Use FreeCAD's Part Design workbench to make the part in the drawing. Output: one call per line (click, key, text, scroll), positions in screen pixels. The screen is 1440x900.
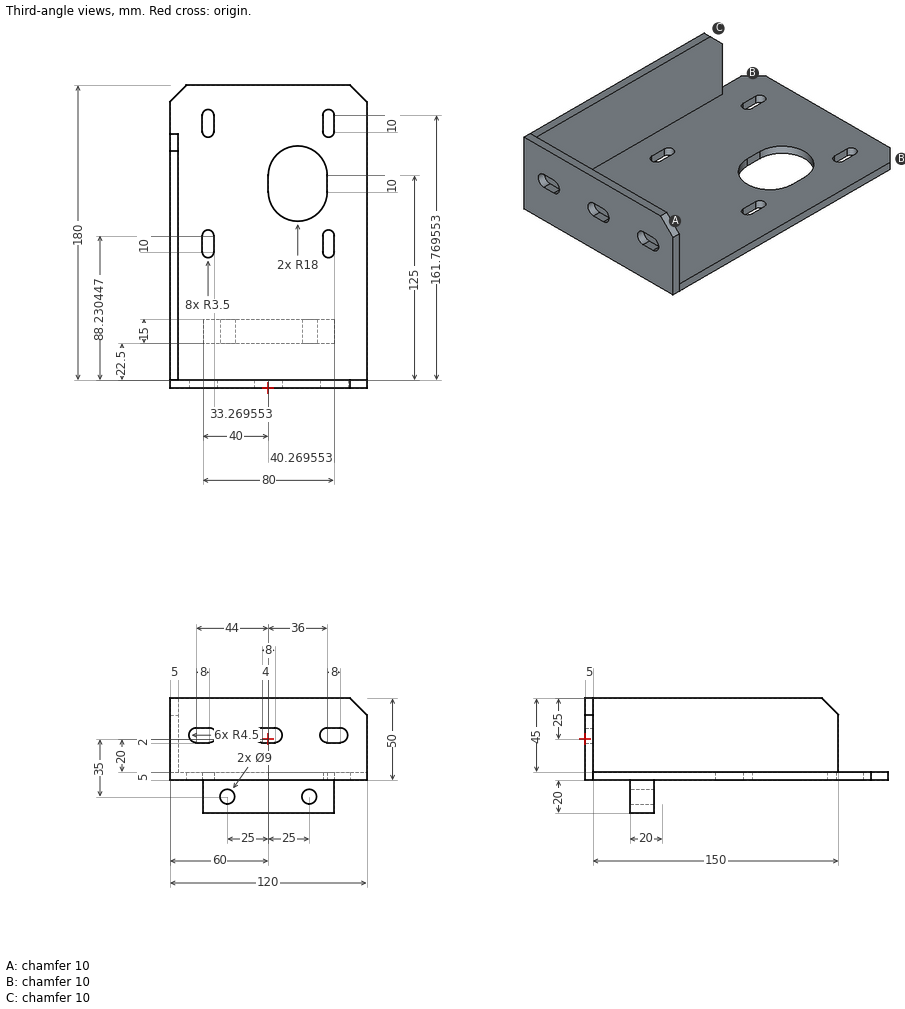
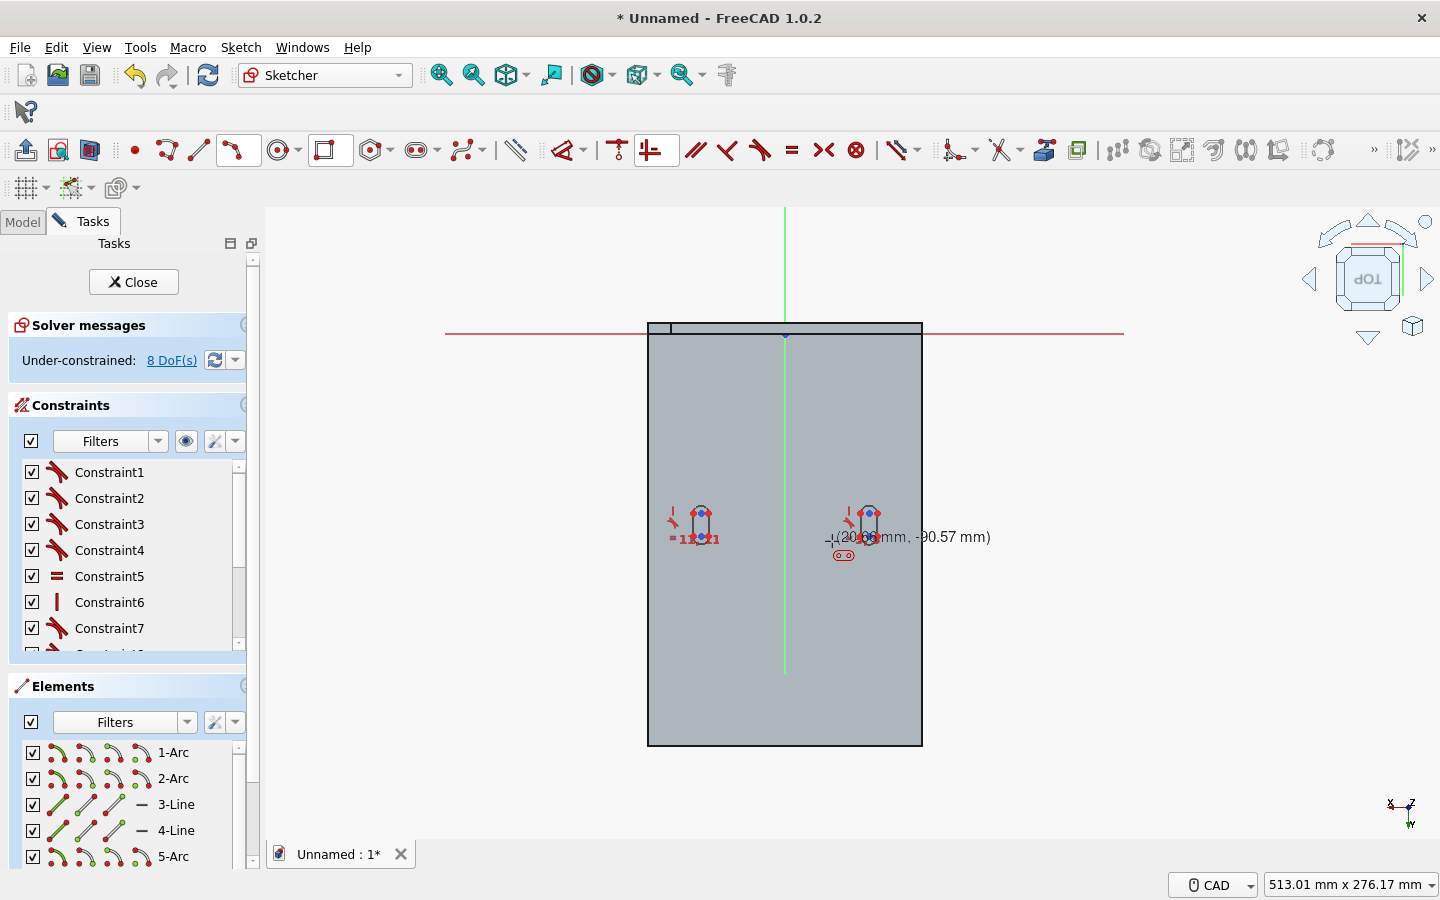
scroll(701, 705, up, 6)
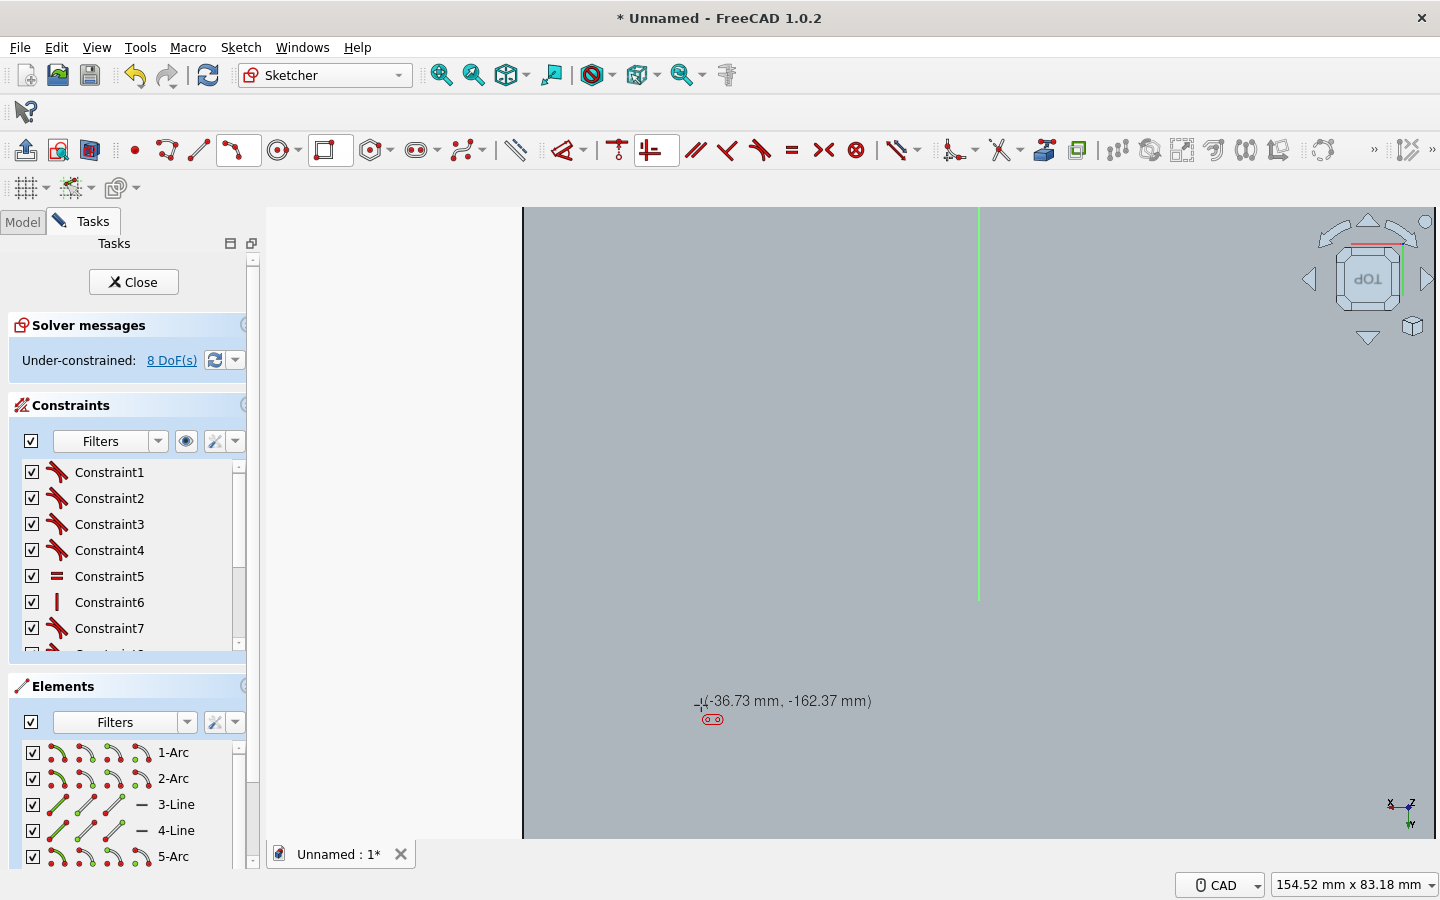
click(700, 702)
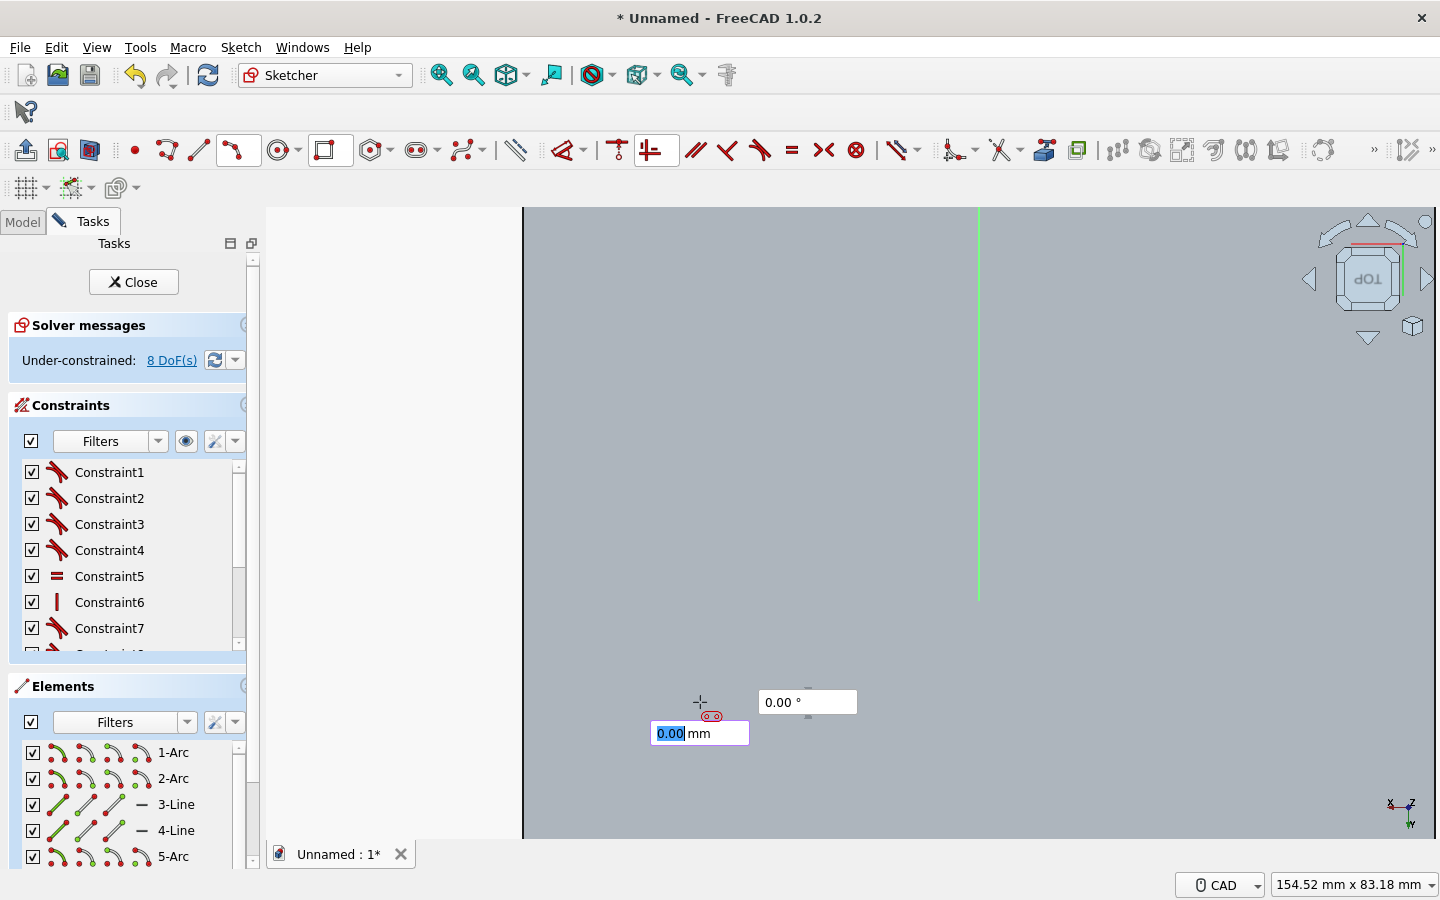
click(700, 626)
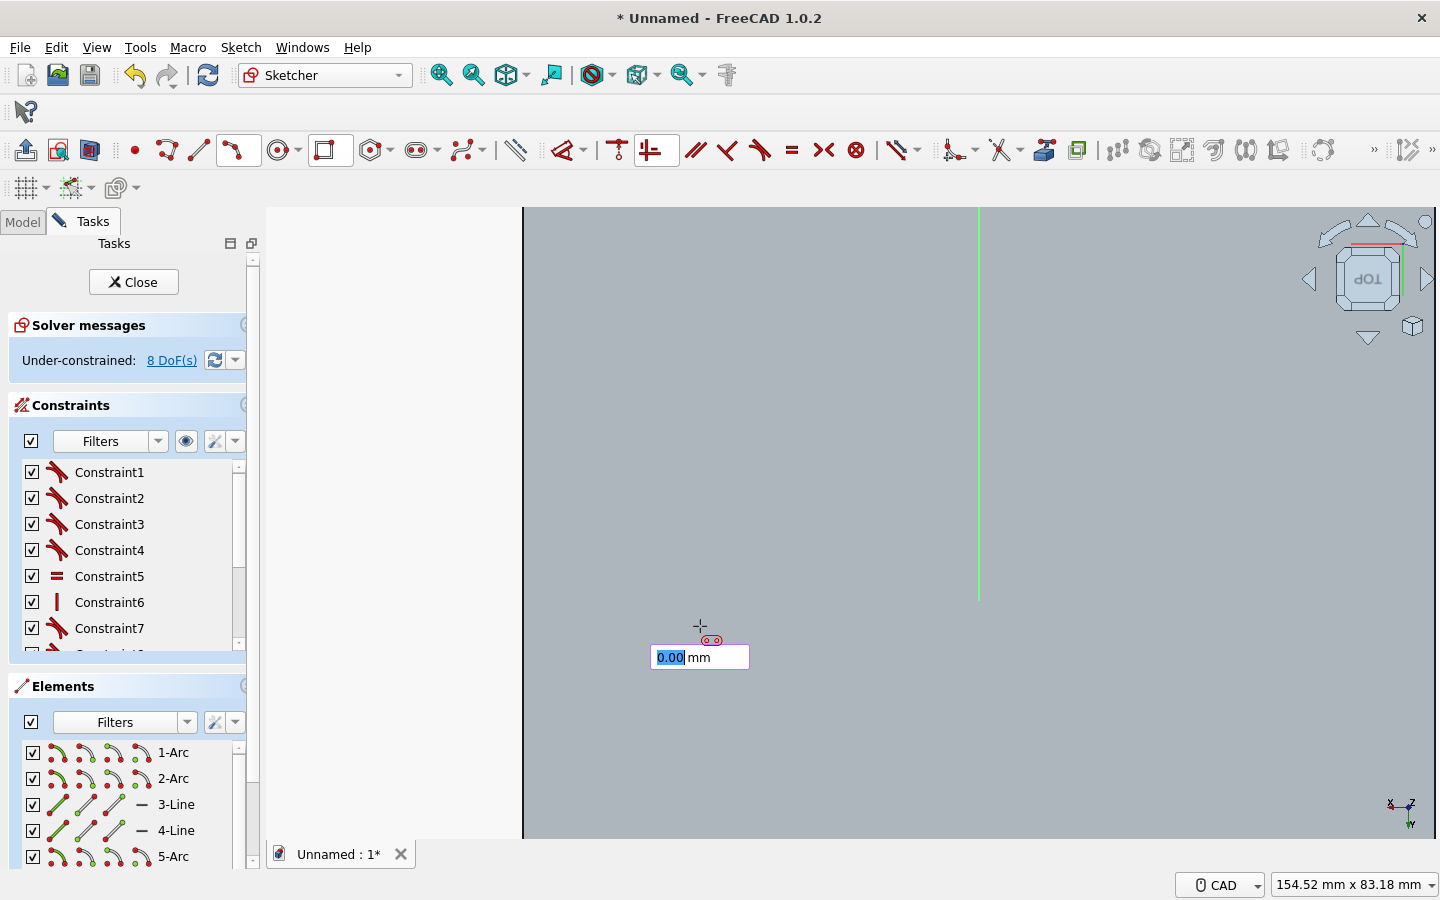
click(726, 664)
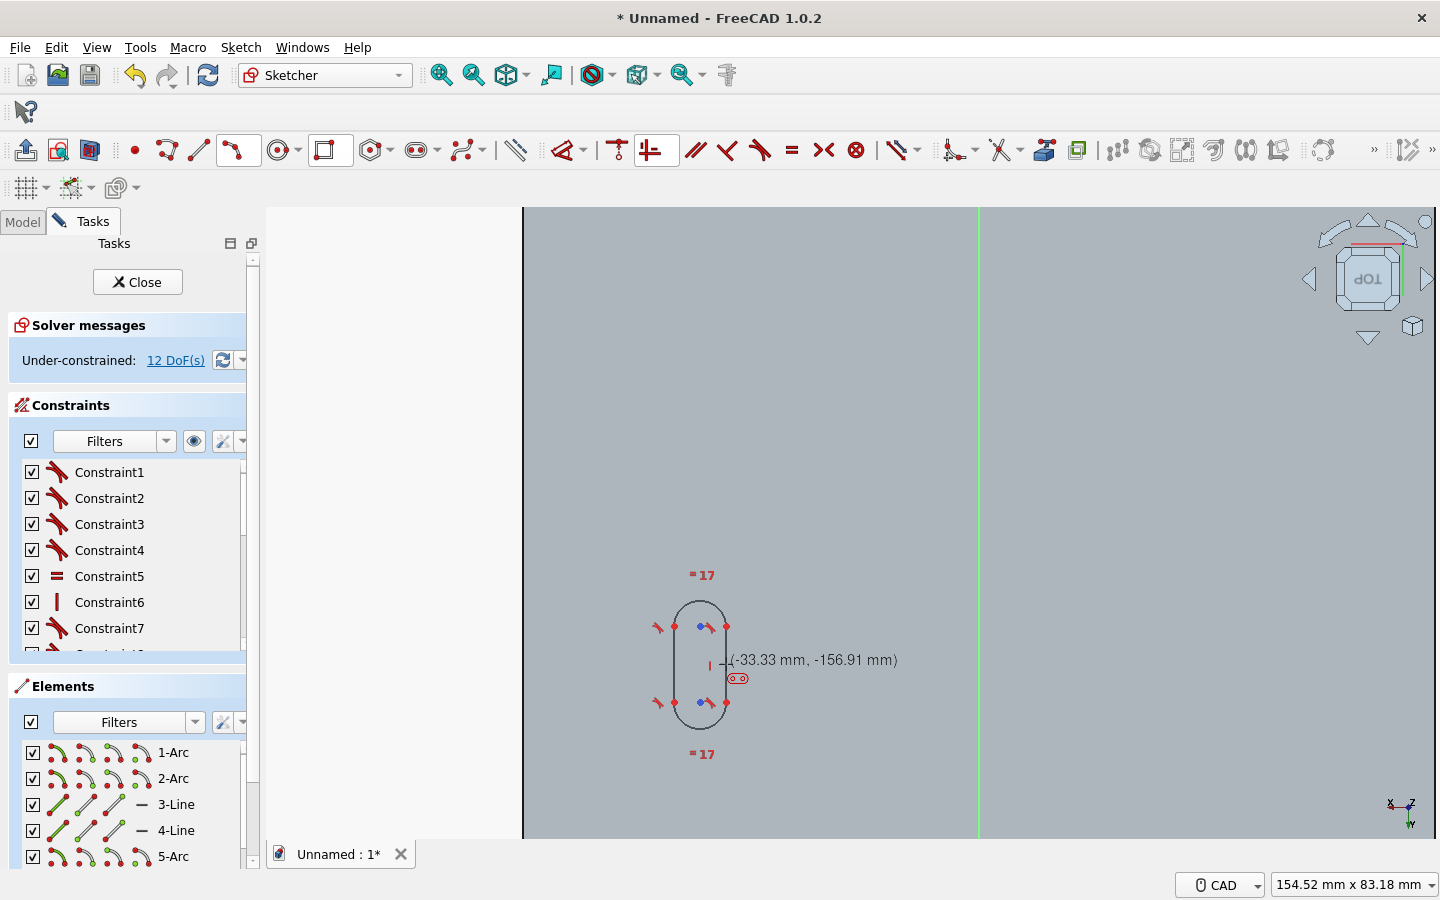
click(1259, 702)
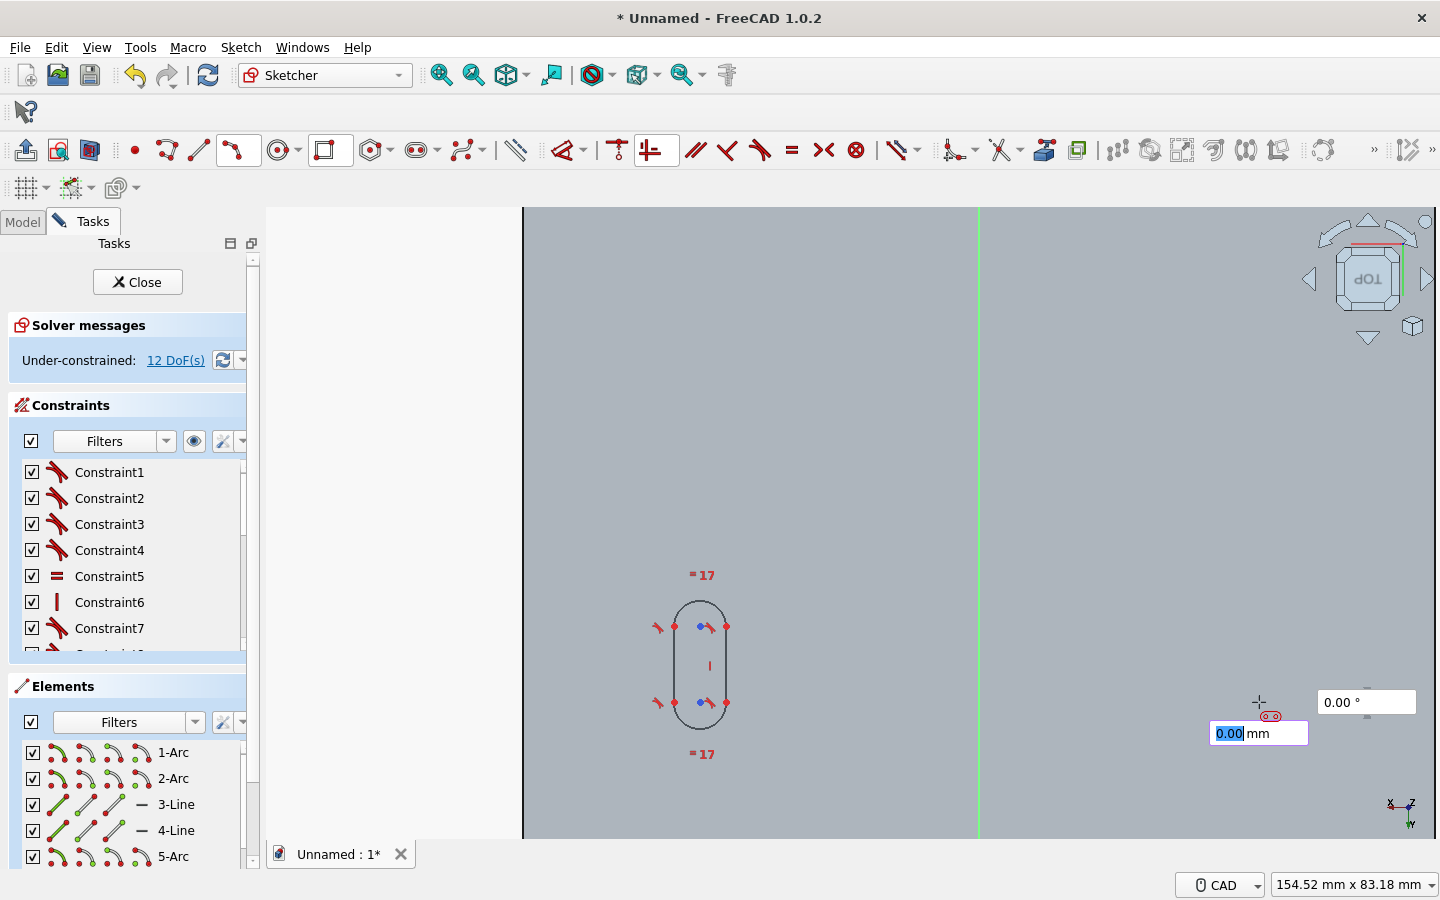
click(1259, 626)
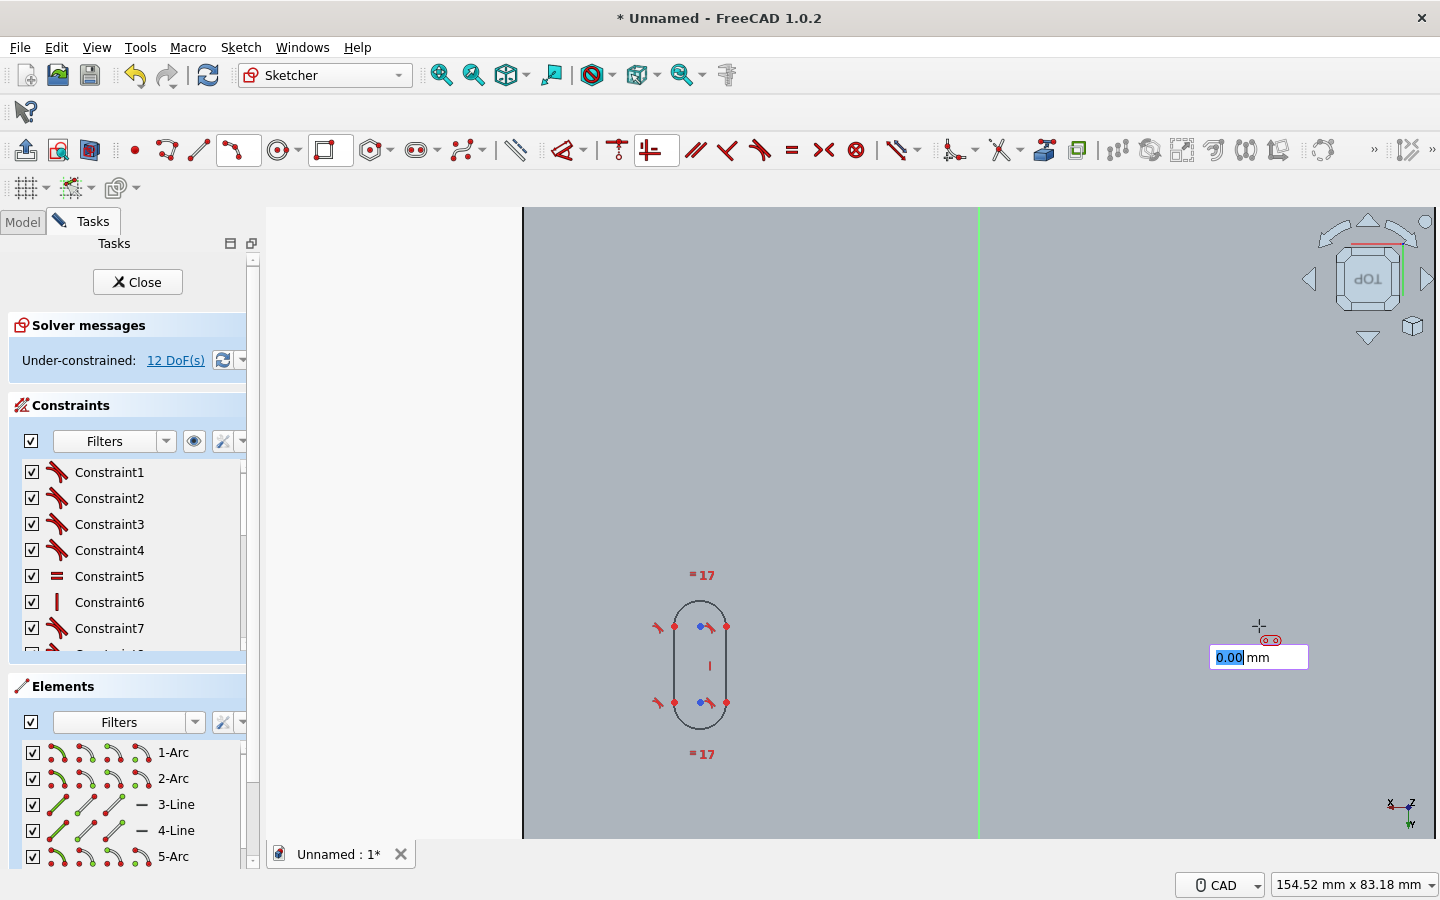
scroll(701, 705, down, 6)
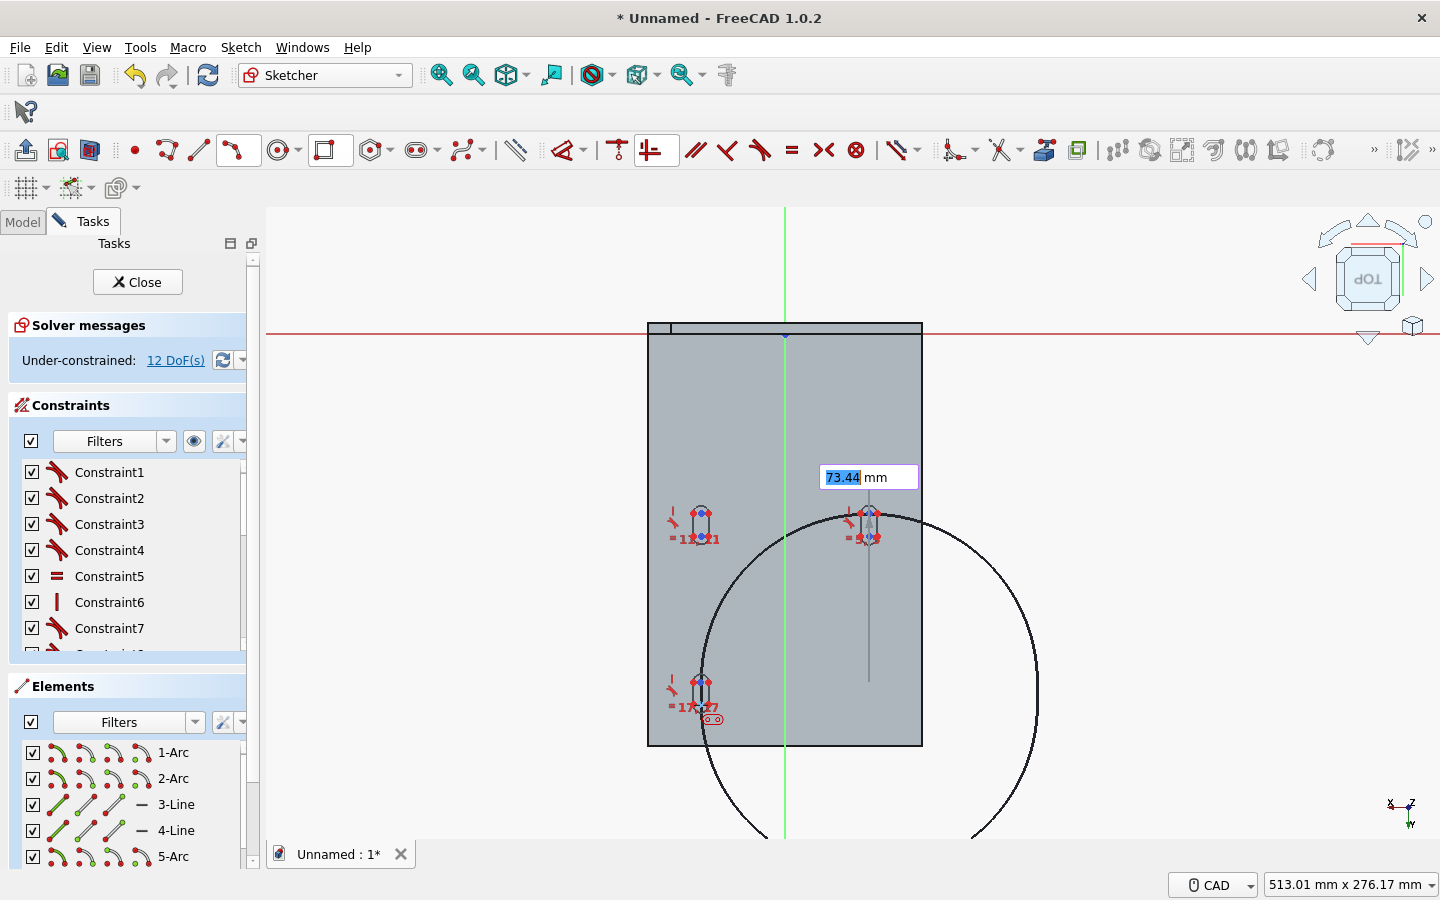
scroll(877, 693, up, 4)